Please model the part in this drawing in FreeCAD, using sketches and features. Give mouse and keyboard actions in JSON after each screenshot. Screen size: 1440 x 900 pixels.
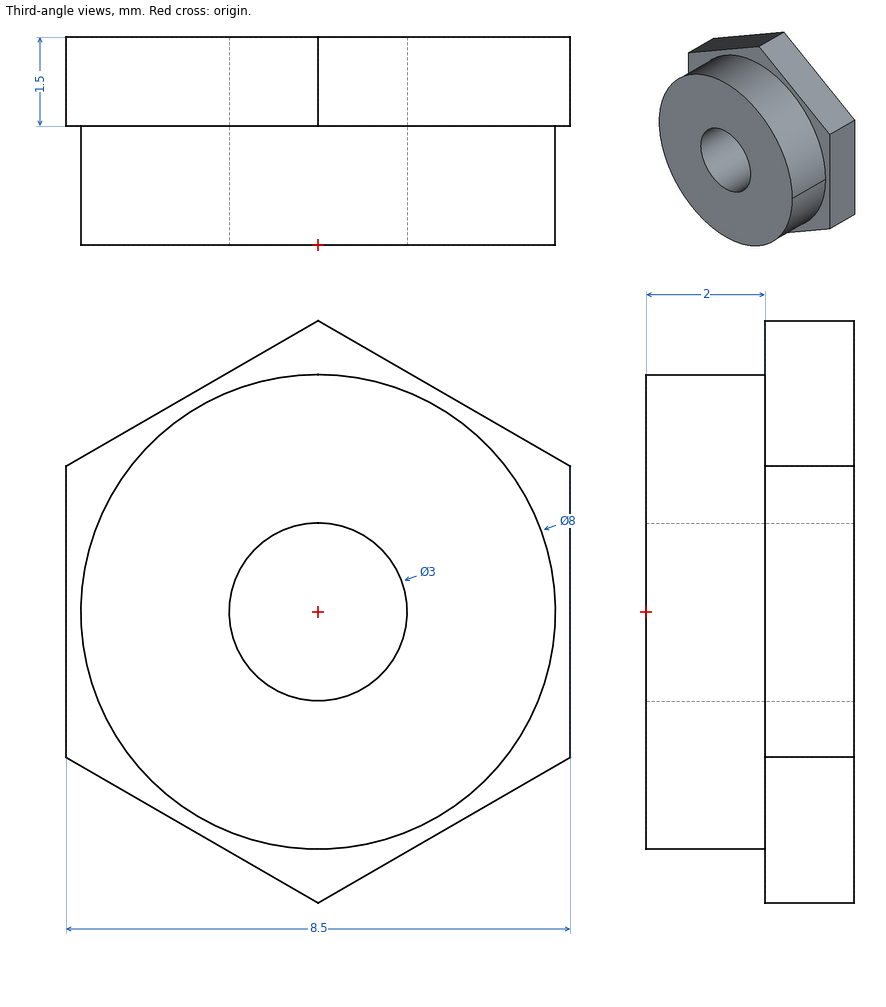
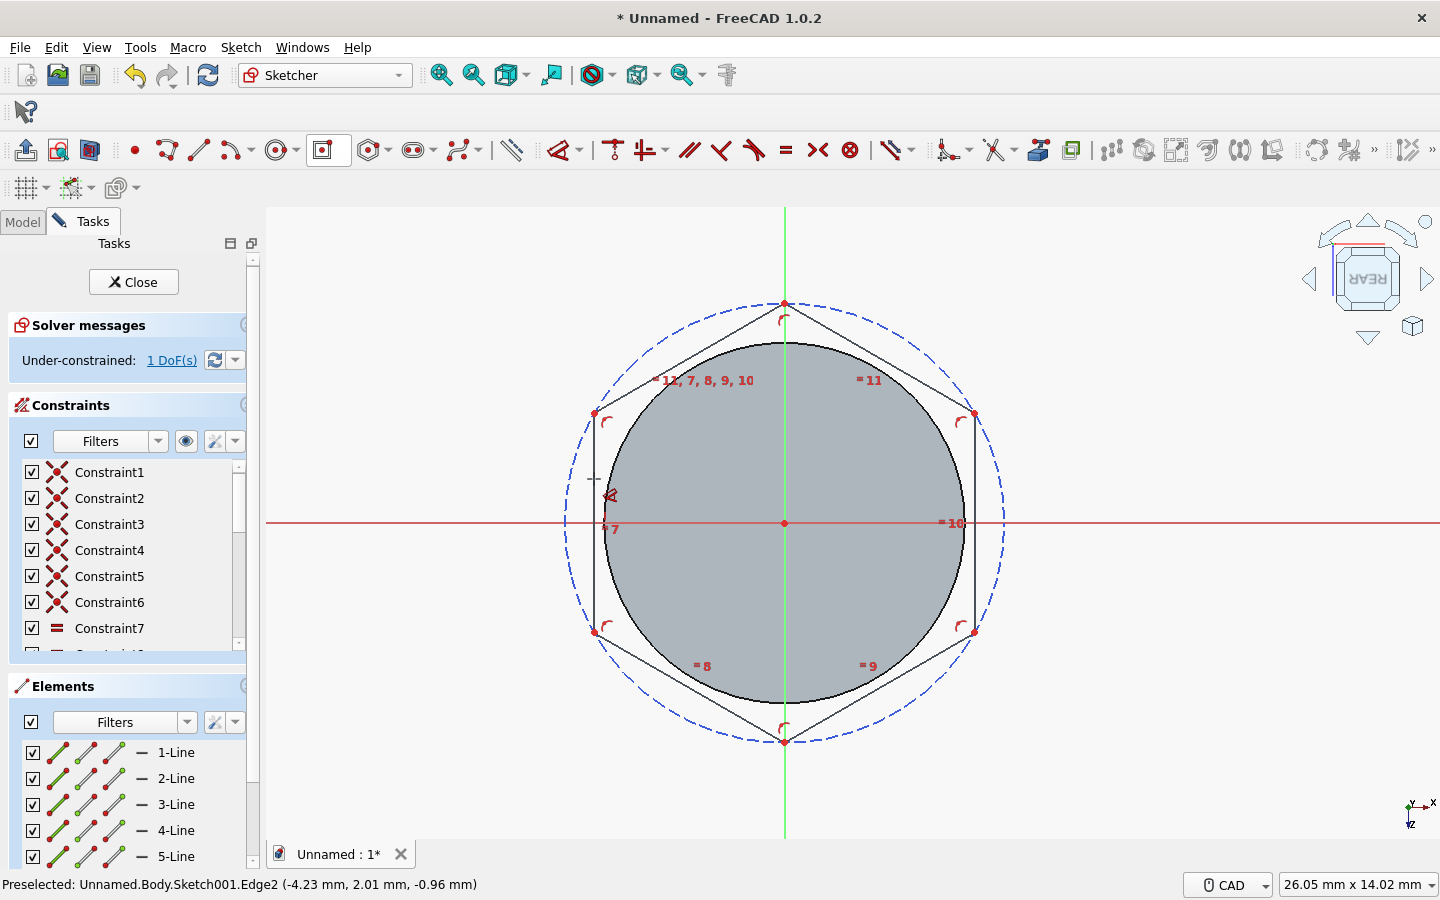
{"action": "left_click", "coordinate": [594, 413]}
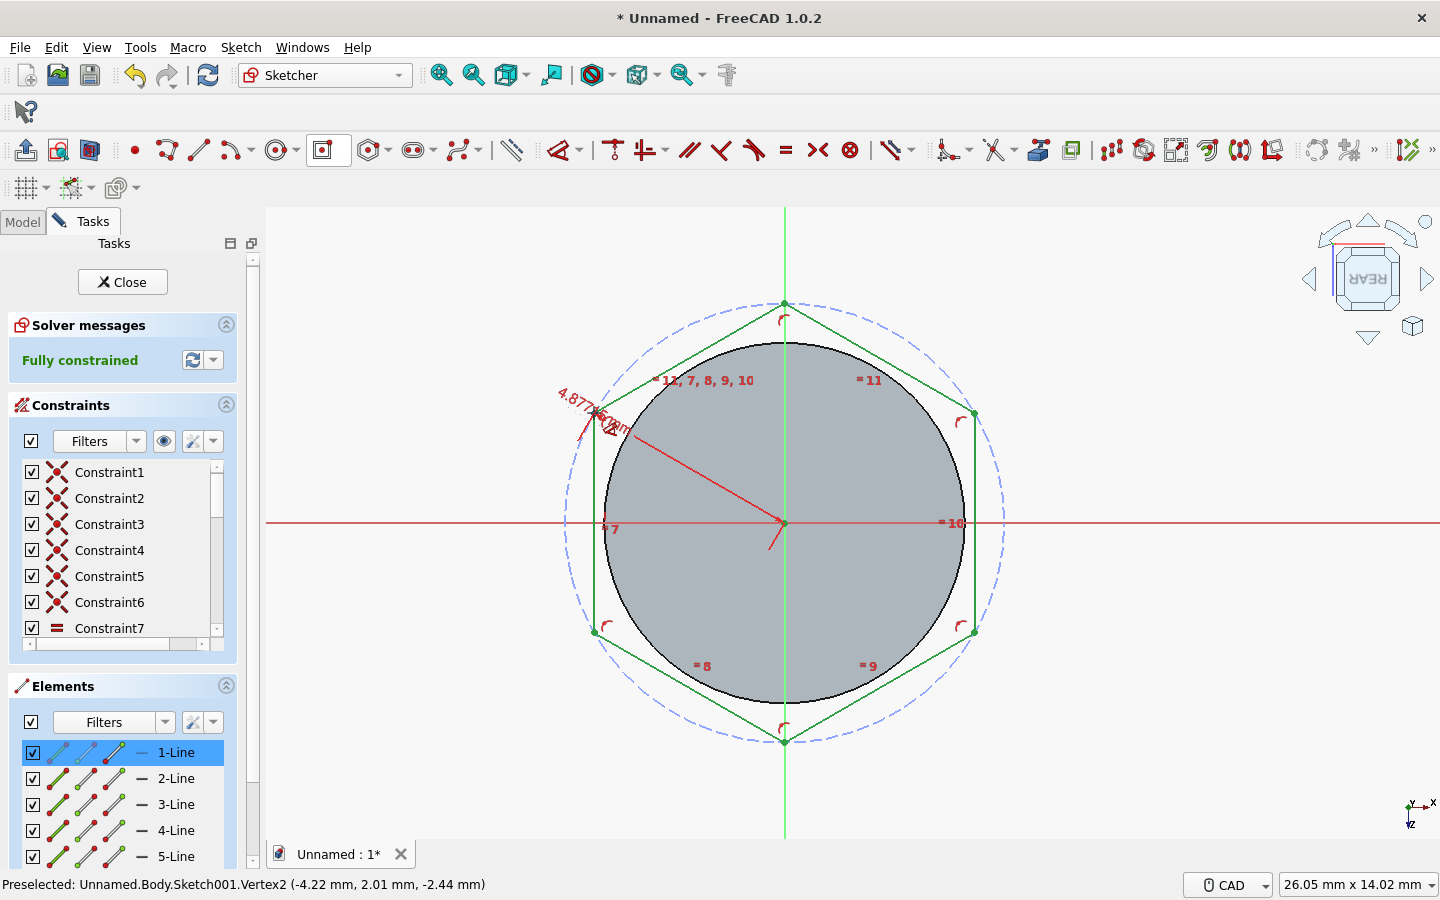
{"action": "left_click", "coordinate": [975, 633]}
{"action": "left_click", "coordinate": [697, 667]}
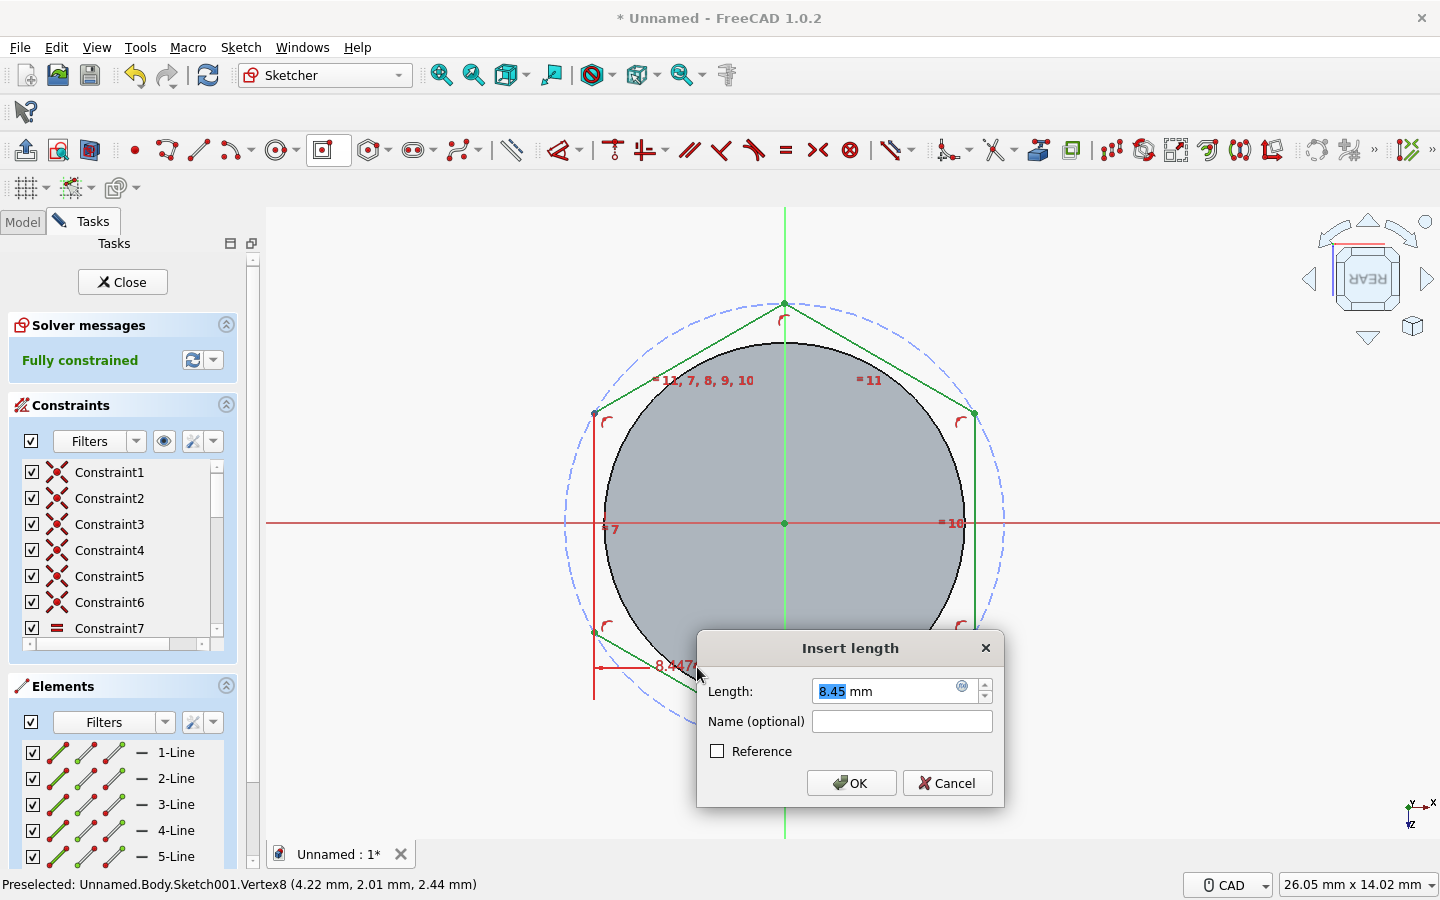
{"action": "type", "text": "8.5"}
{"action": "key", "text": "Return"}
{"action": "key", "text": "Escape"}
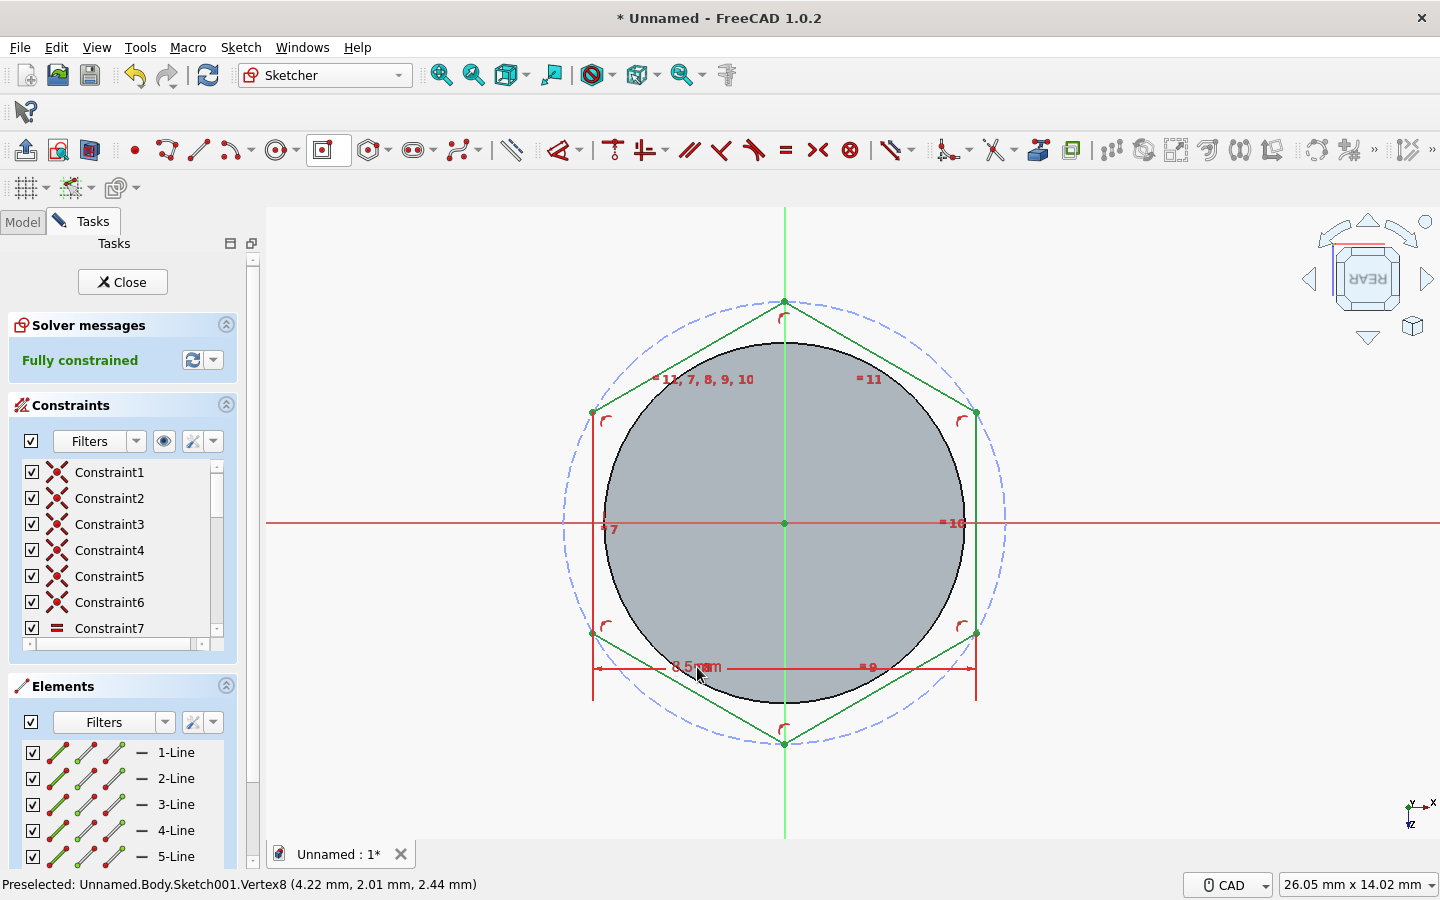
{"action": "left_click", "coordinate": [123, 282]}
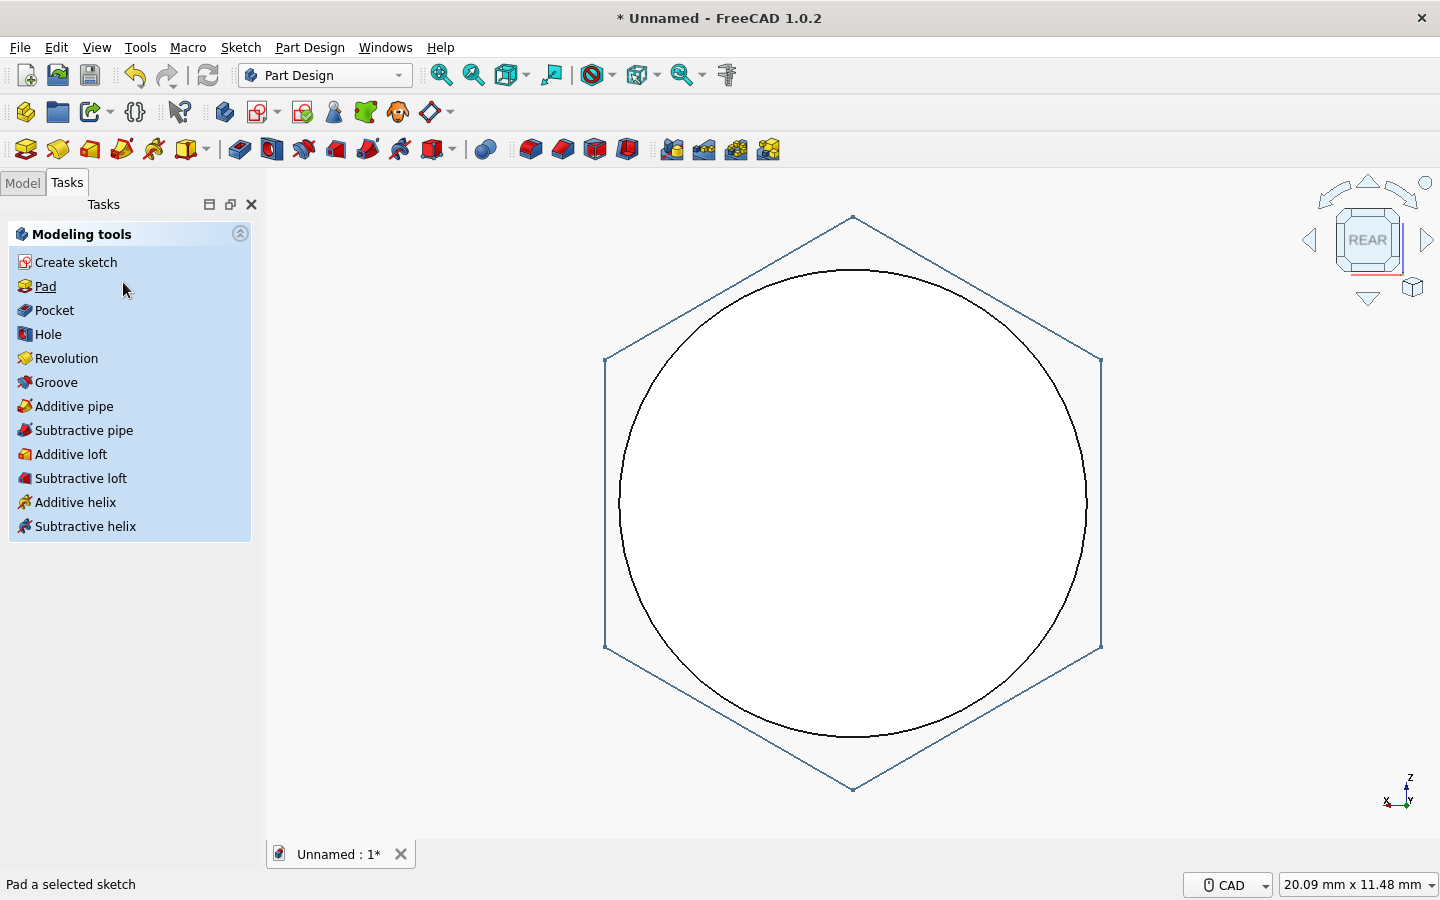
{"action": "left_click", "coordinate": [26, 150]}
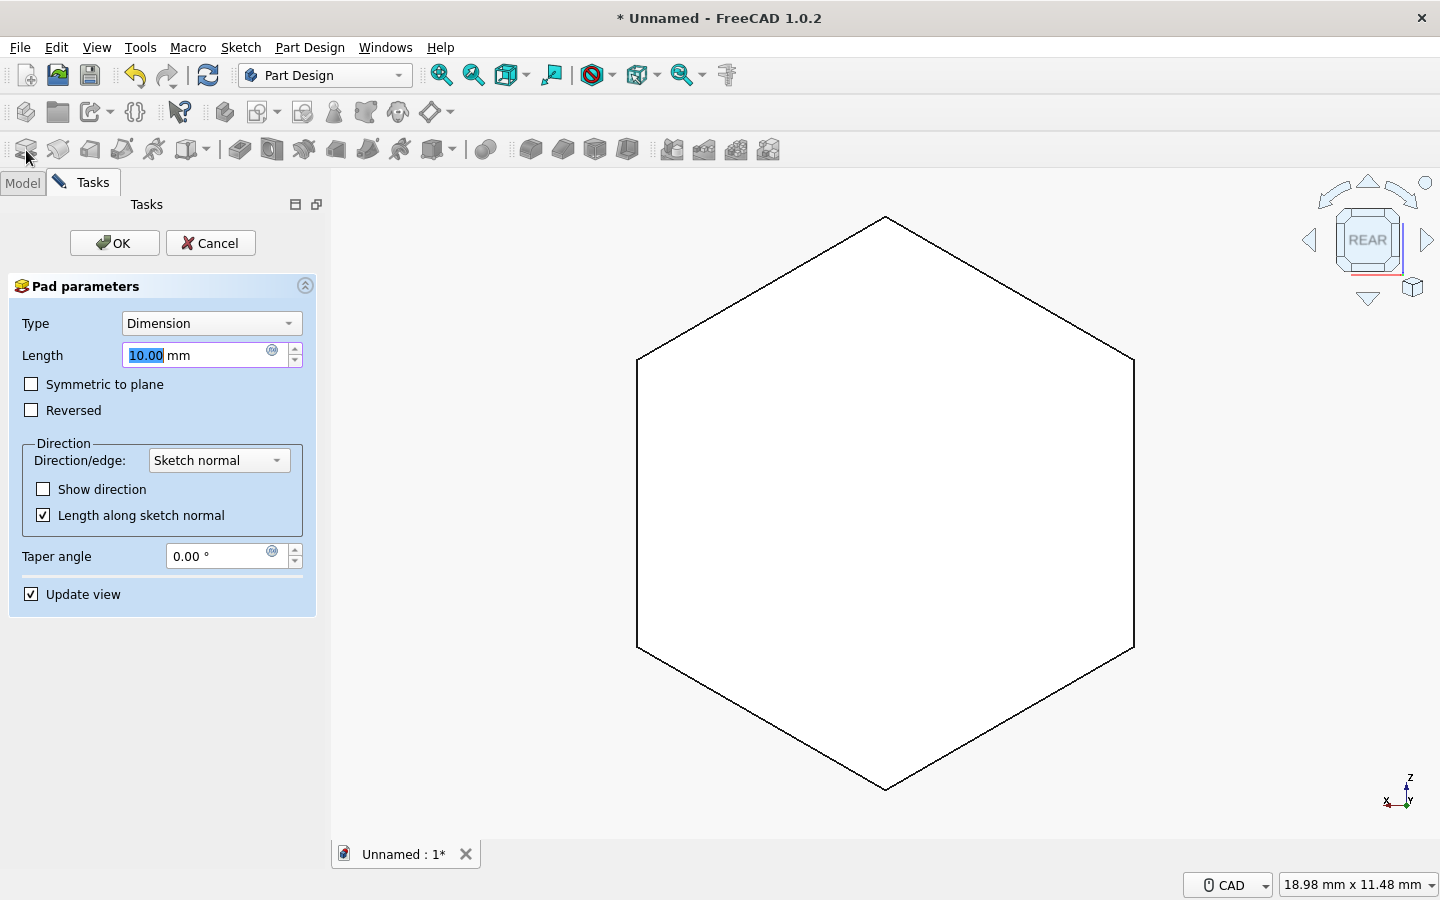
{"action": "type", "text": "1.5"}
{"action": "key", "text": "Tab"}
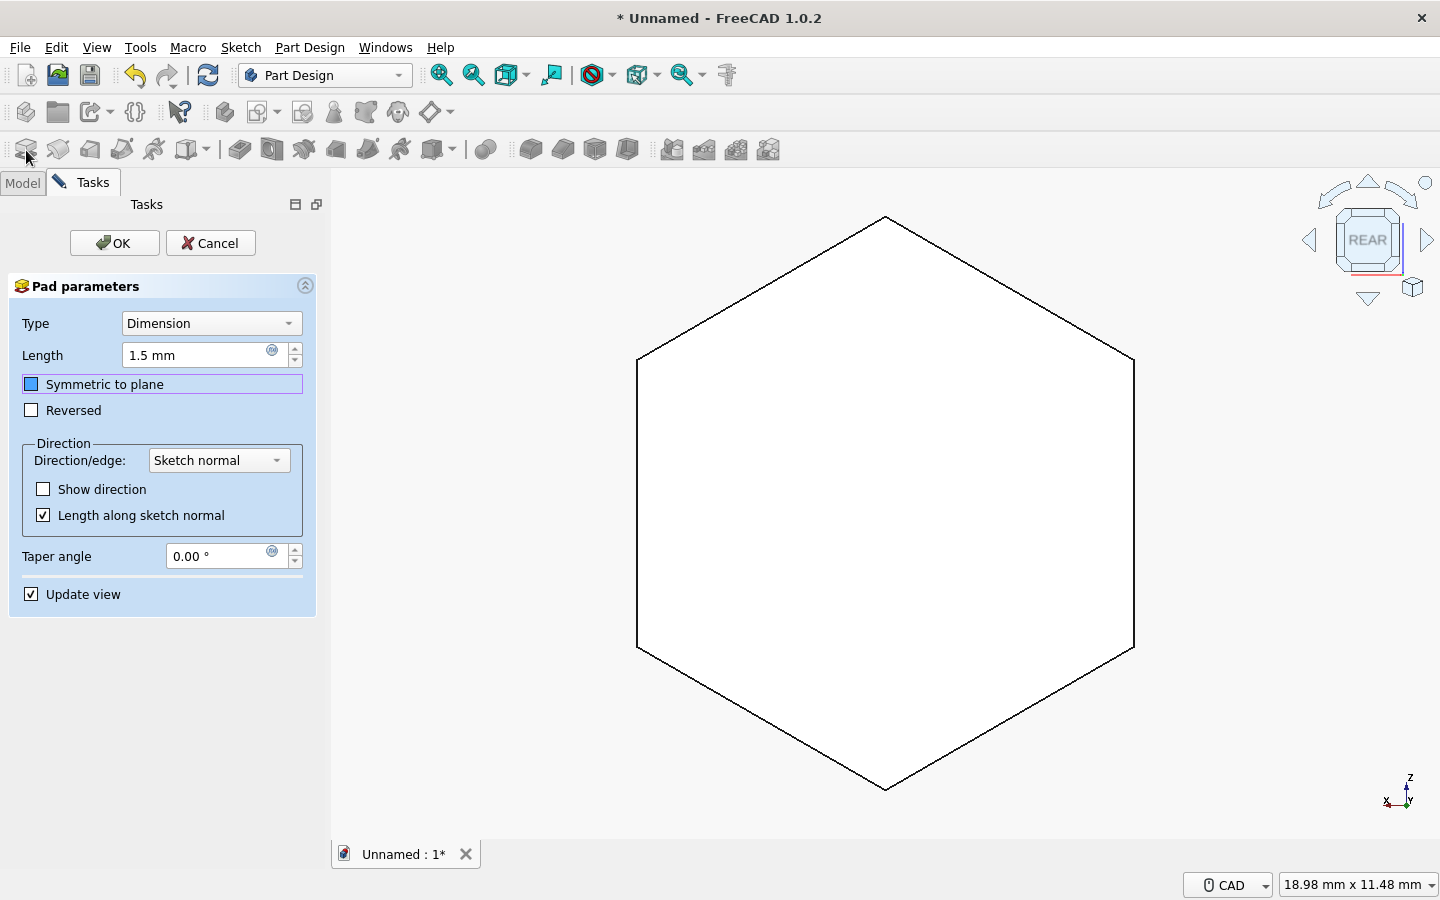
{"action": "left_click", "coordinate": [115, 243]}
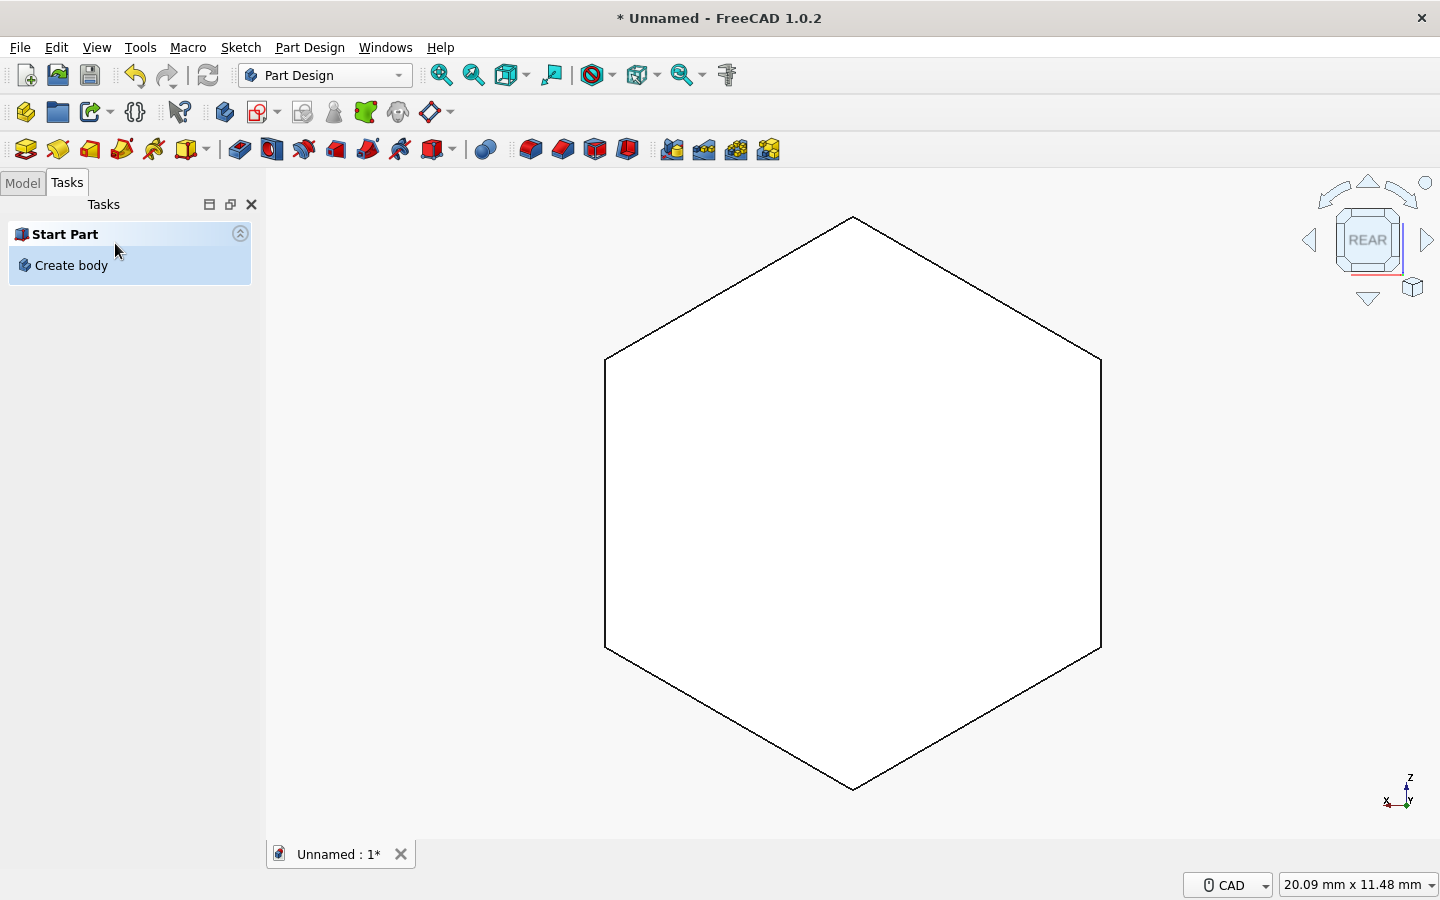
{"action": "left_click", "coordinate": [853, 502]}